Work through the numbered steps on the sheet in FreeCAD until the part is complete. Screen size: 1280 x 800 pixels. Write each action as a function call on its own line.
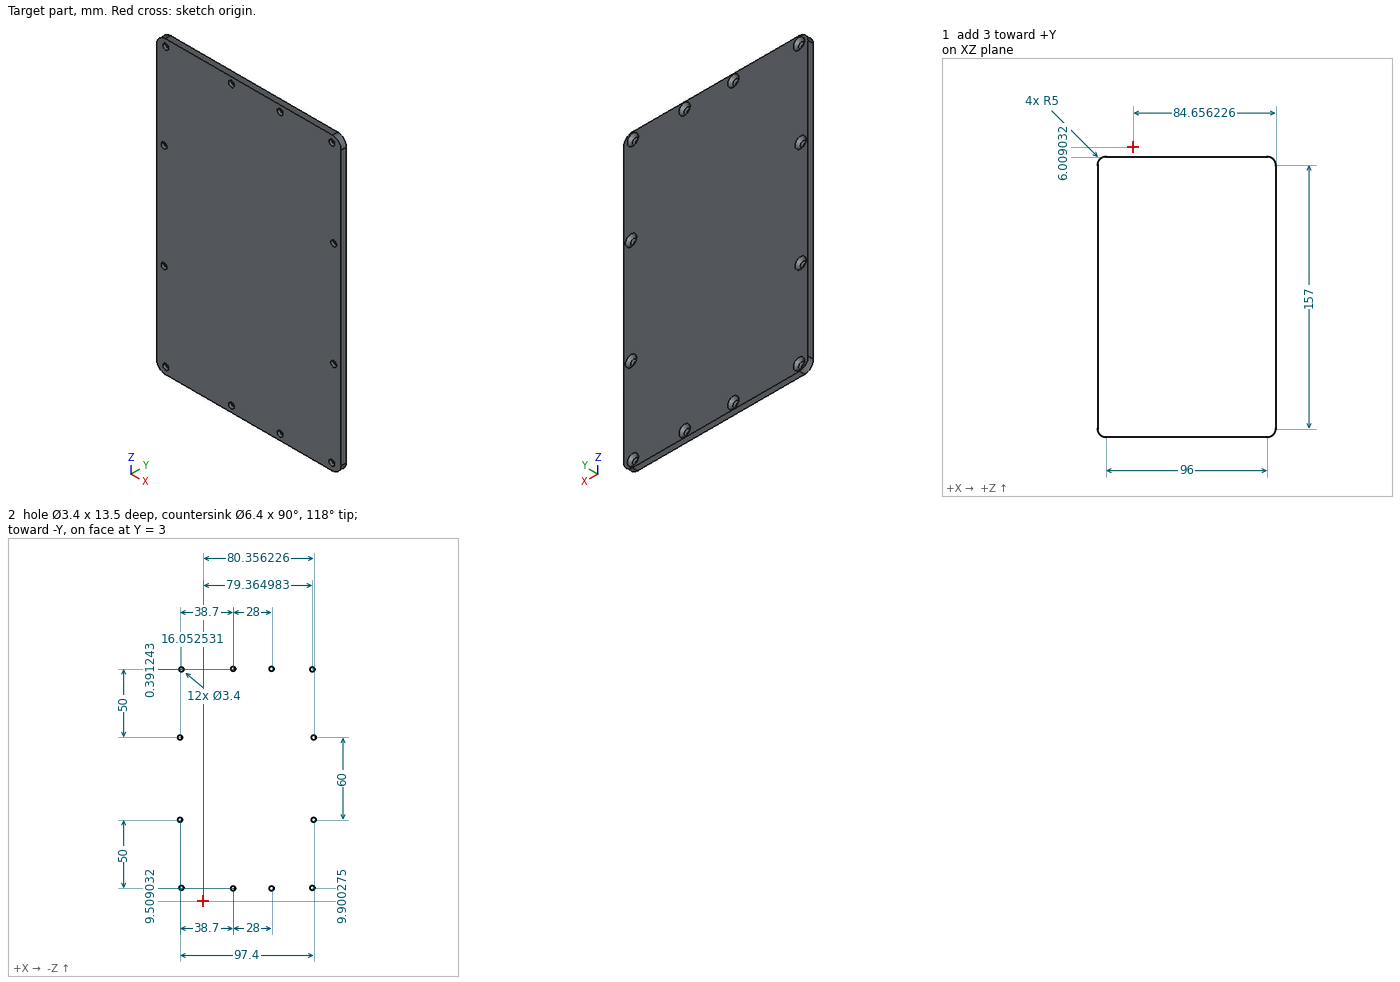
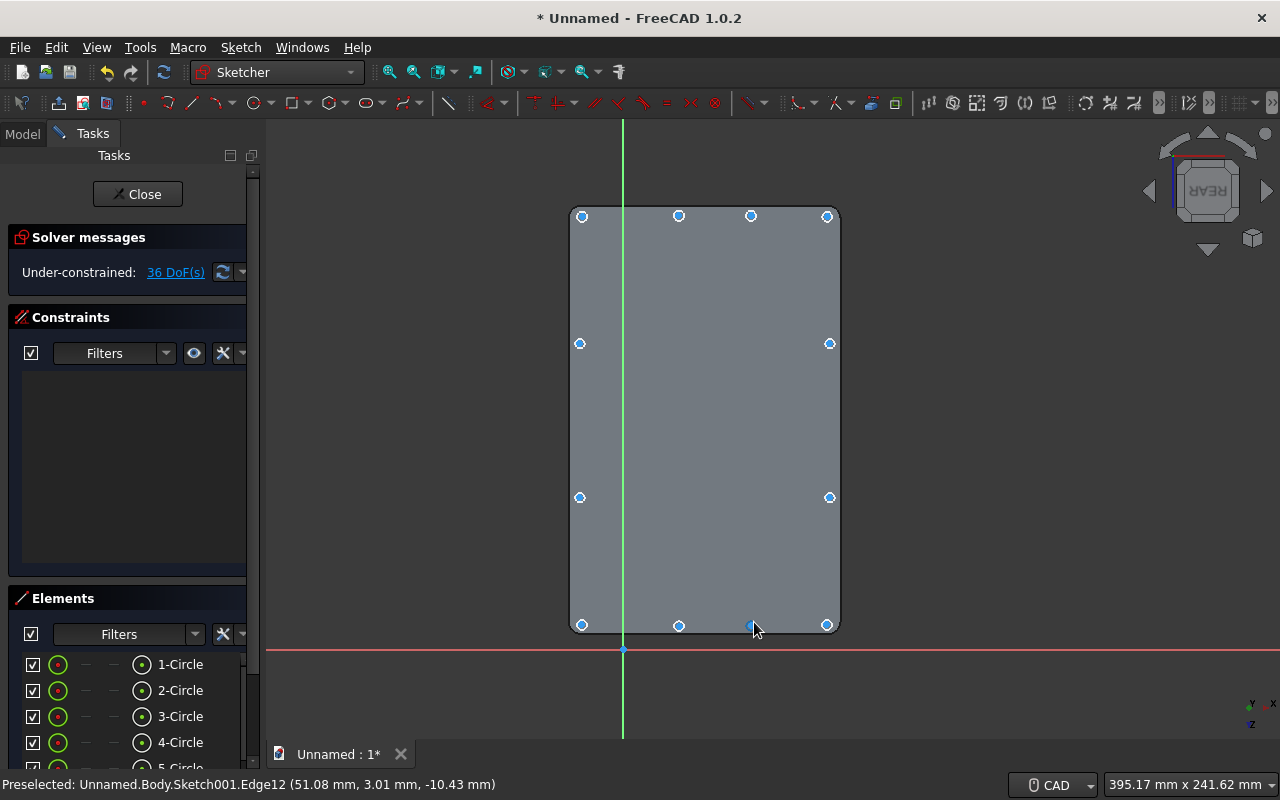
scroll(586, 213, up, 6)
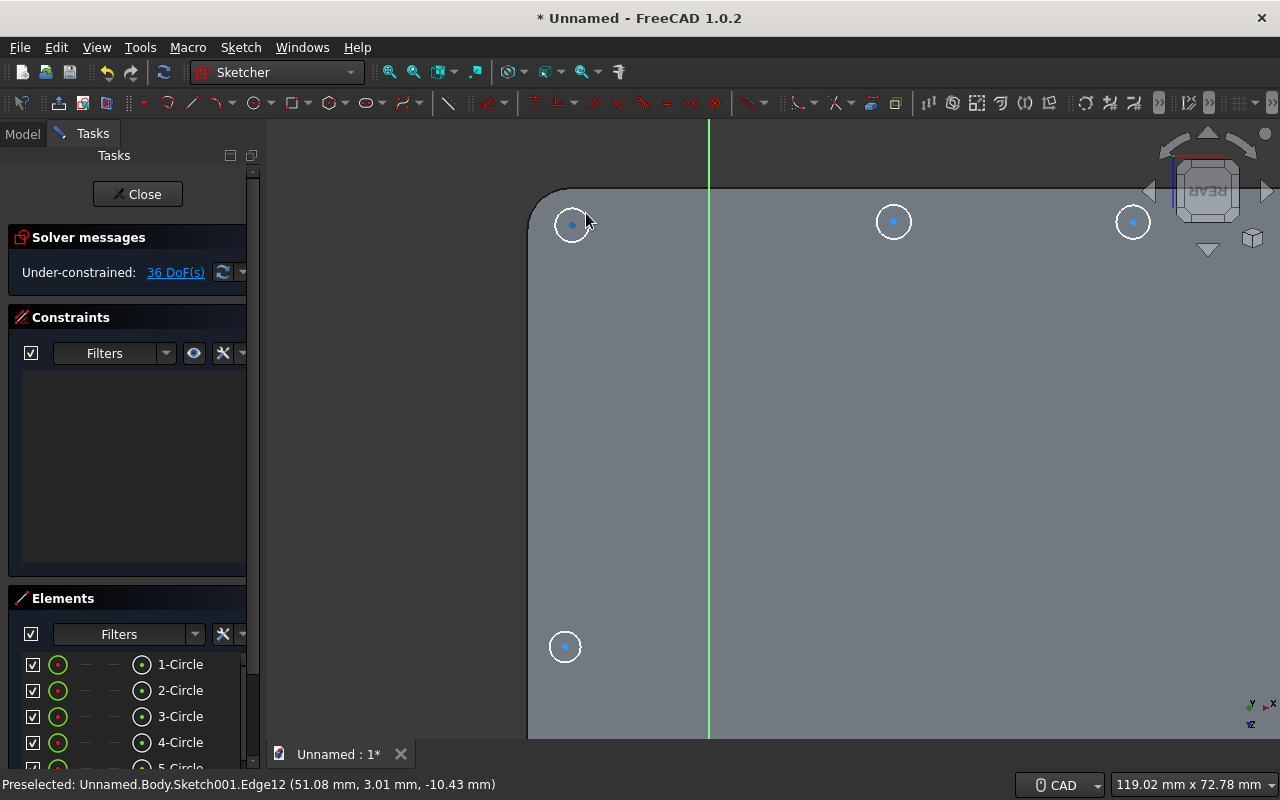
click(584, 213)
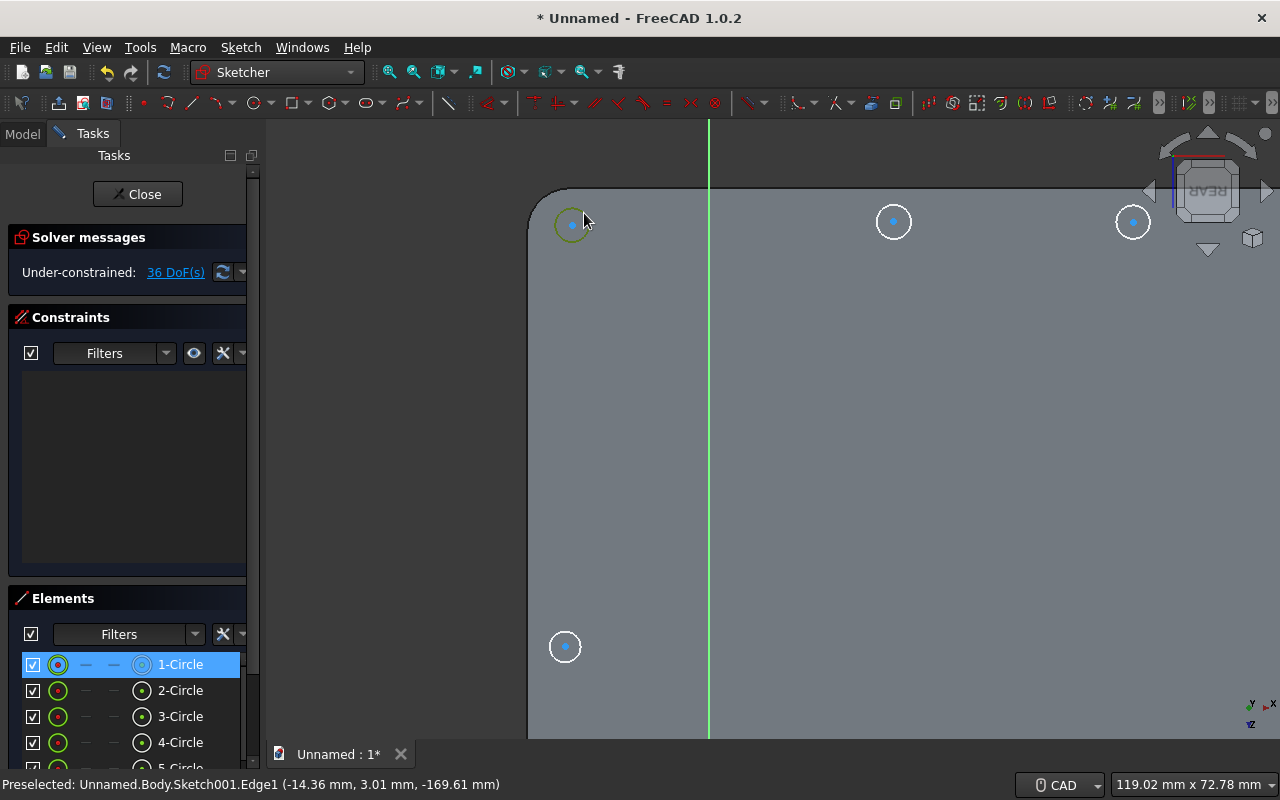
scroll(586, 212, down, 6)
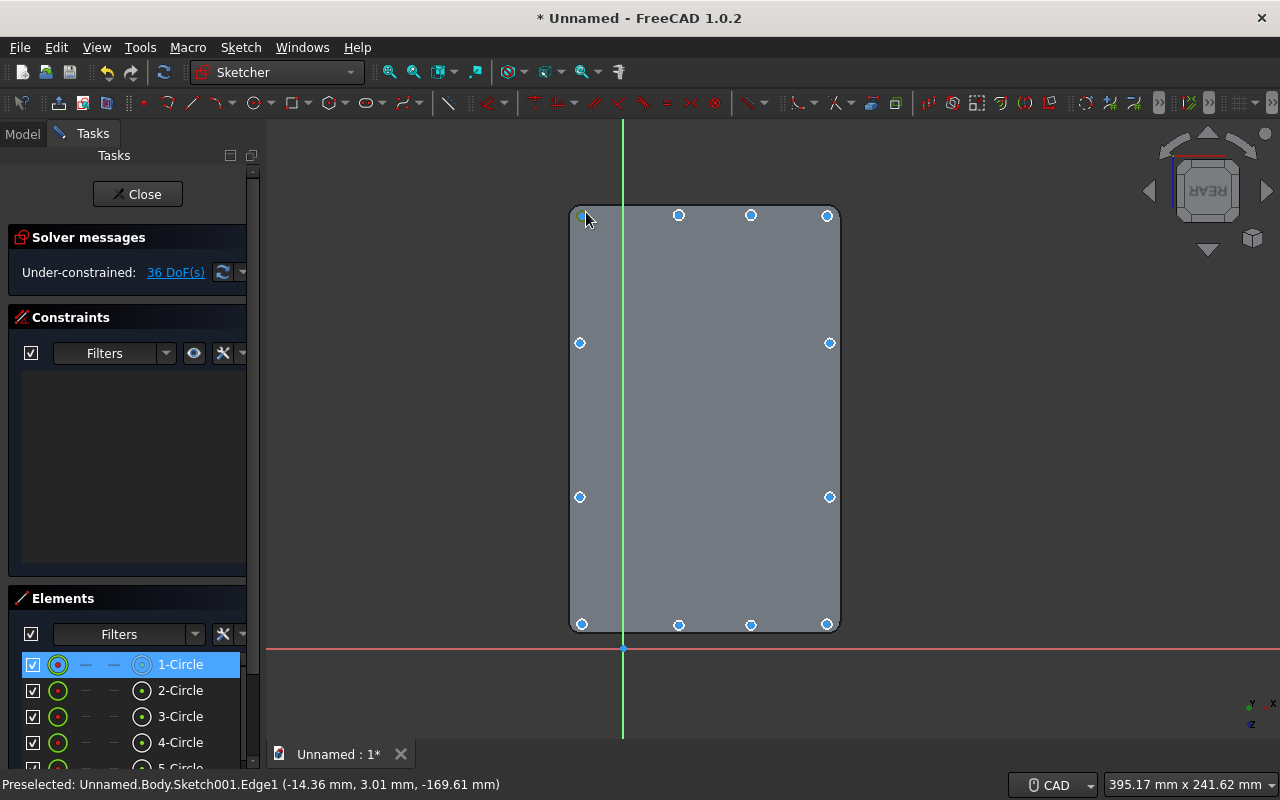
scroll(831, 213, up, 6)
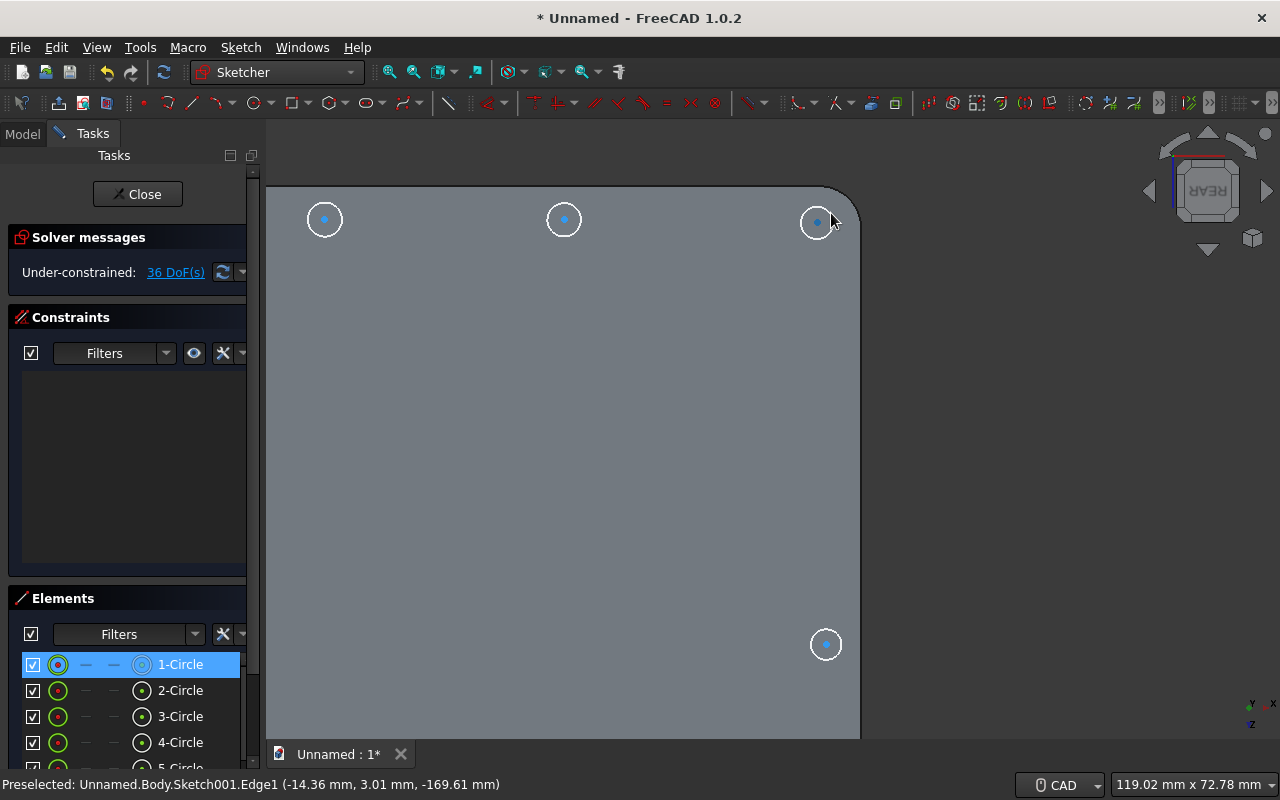
click(828, 211)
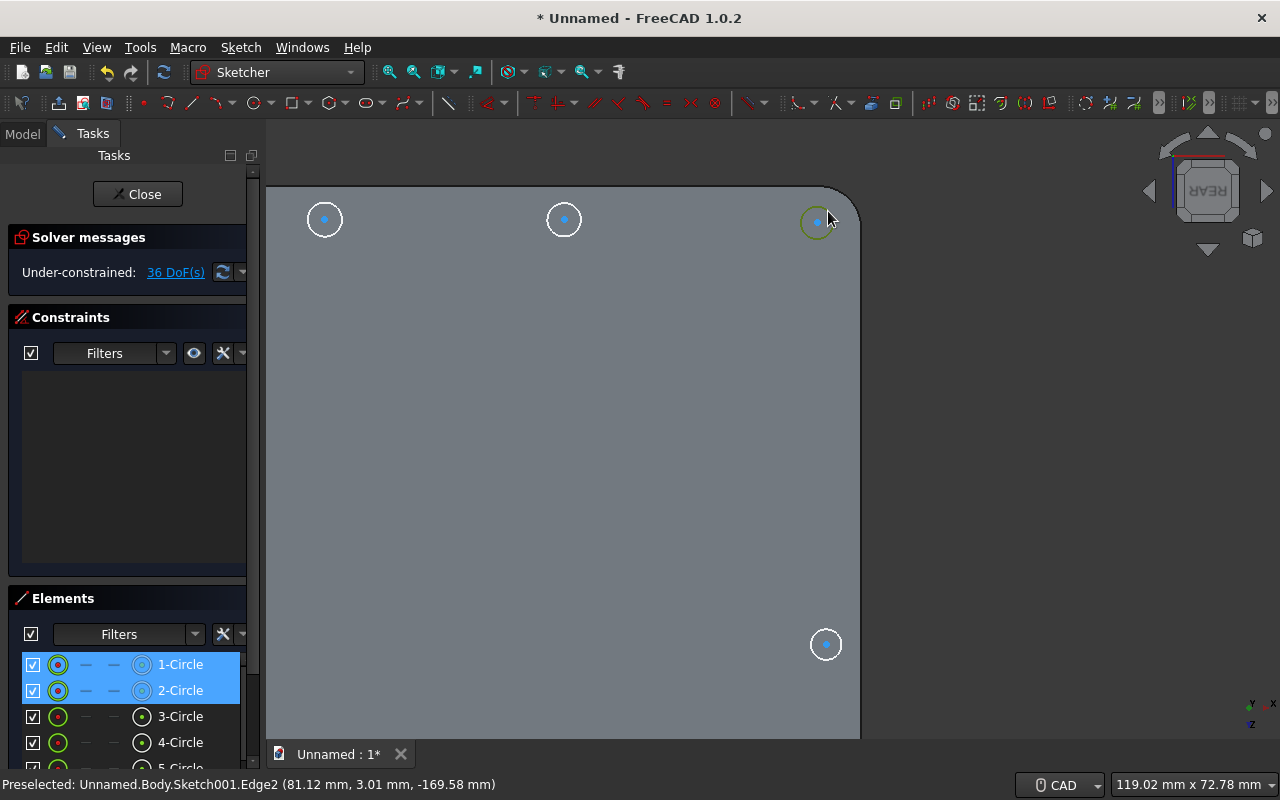
click(837, 634)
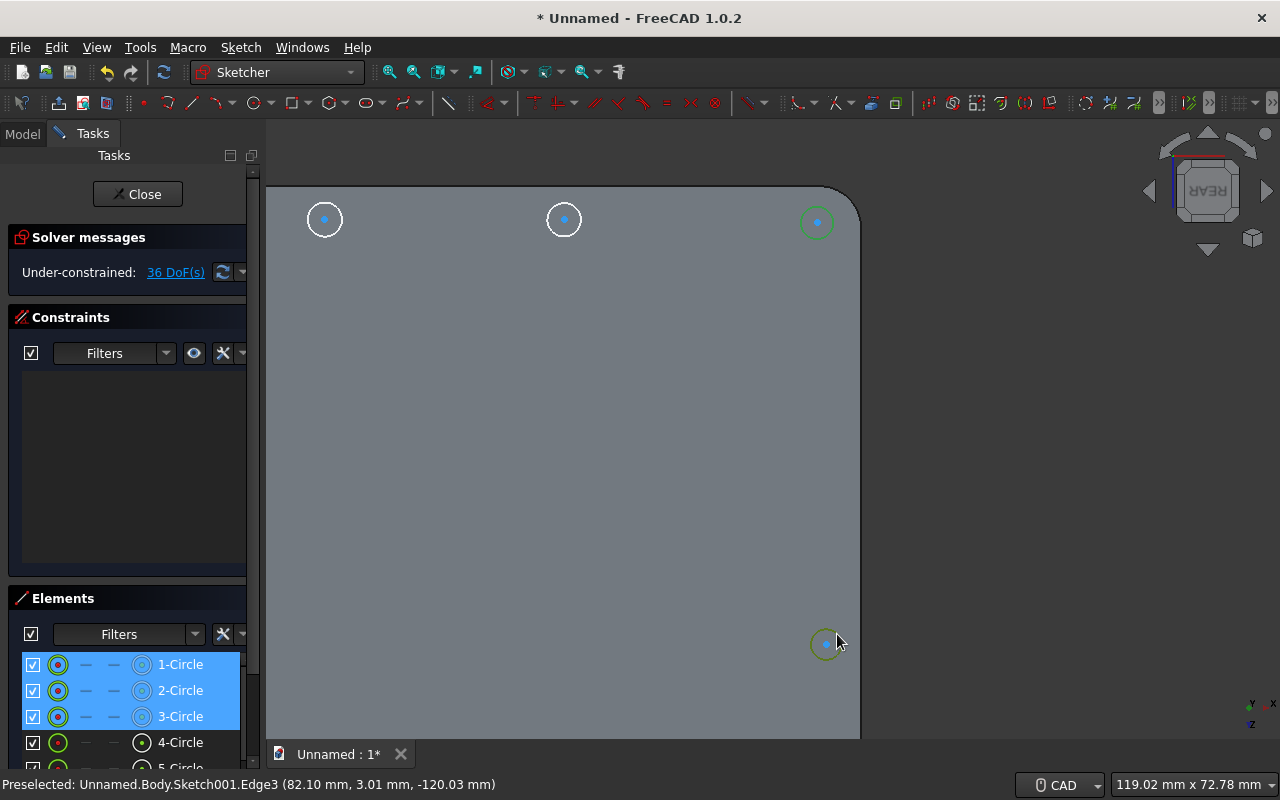
scroll(832, 213, down, 6)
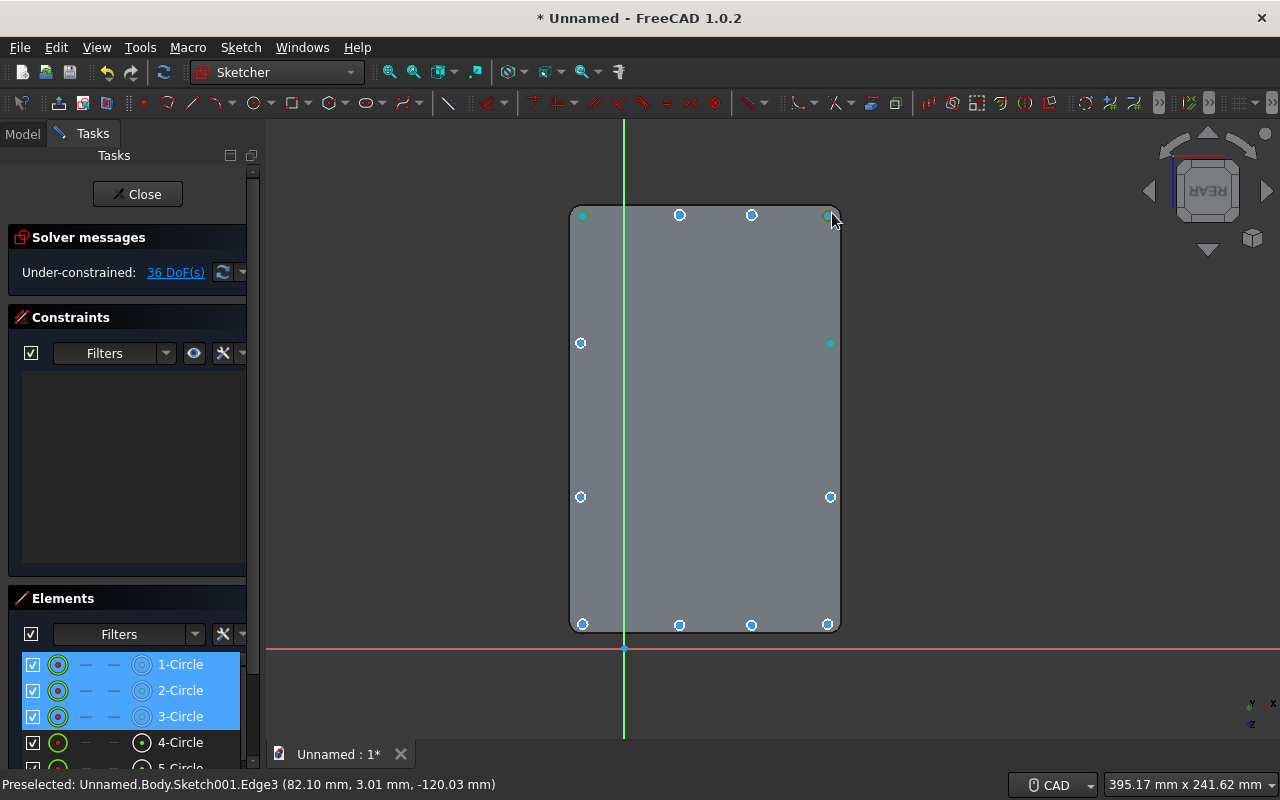
scroll(834, 494, up, 6)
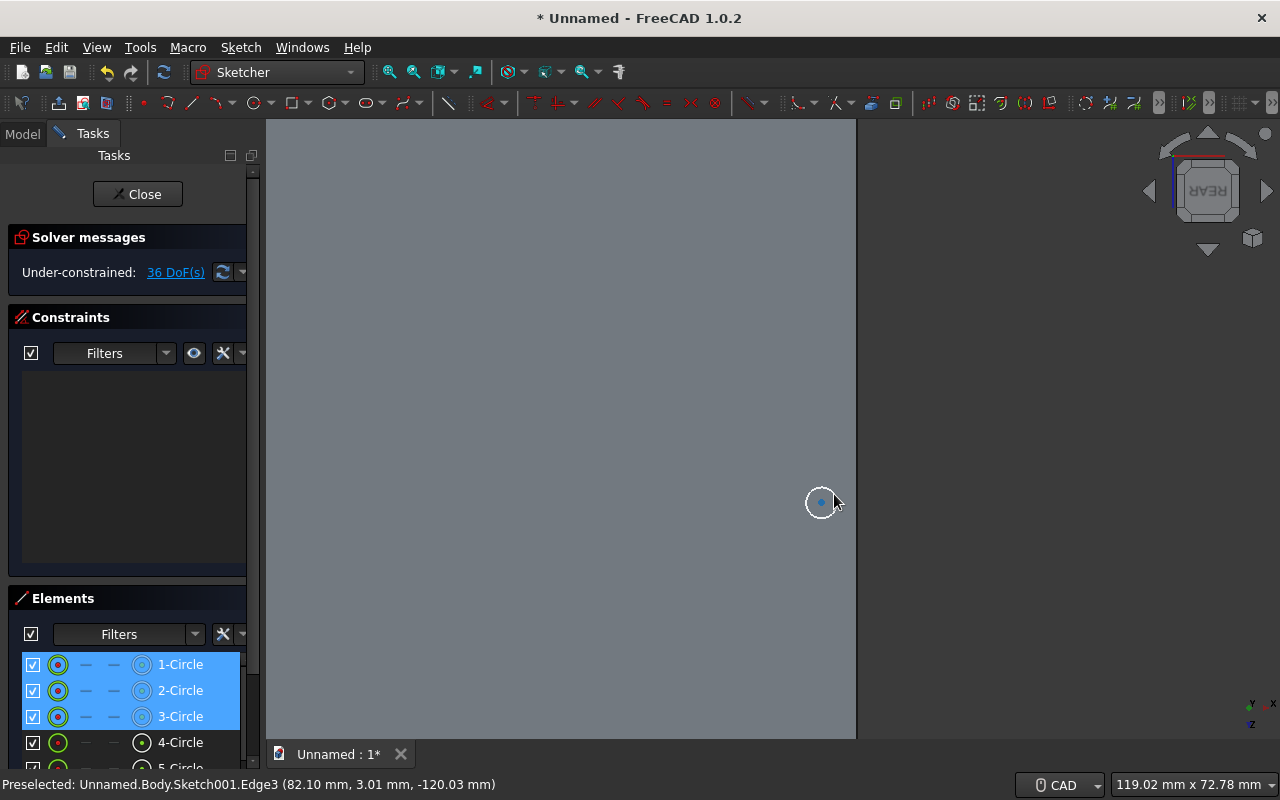
click(832, 492)